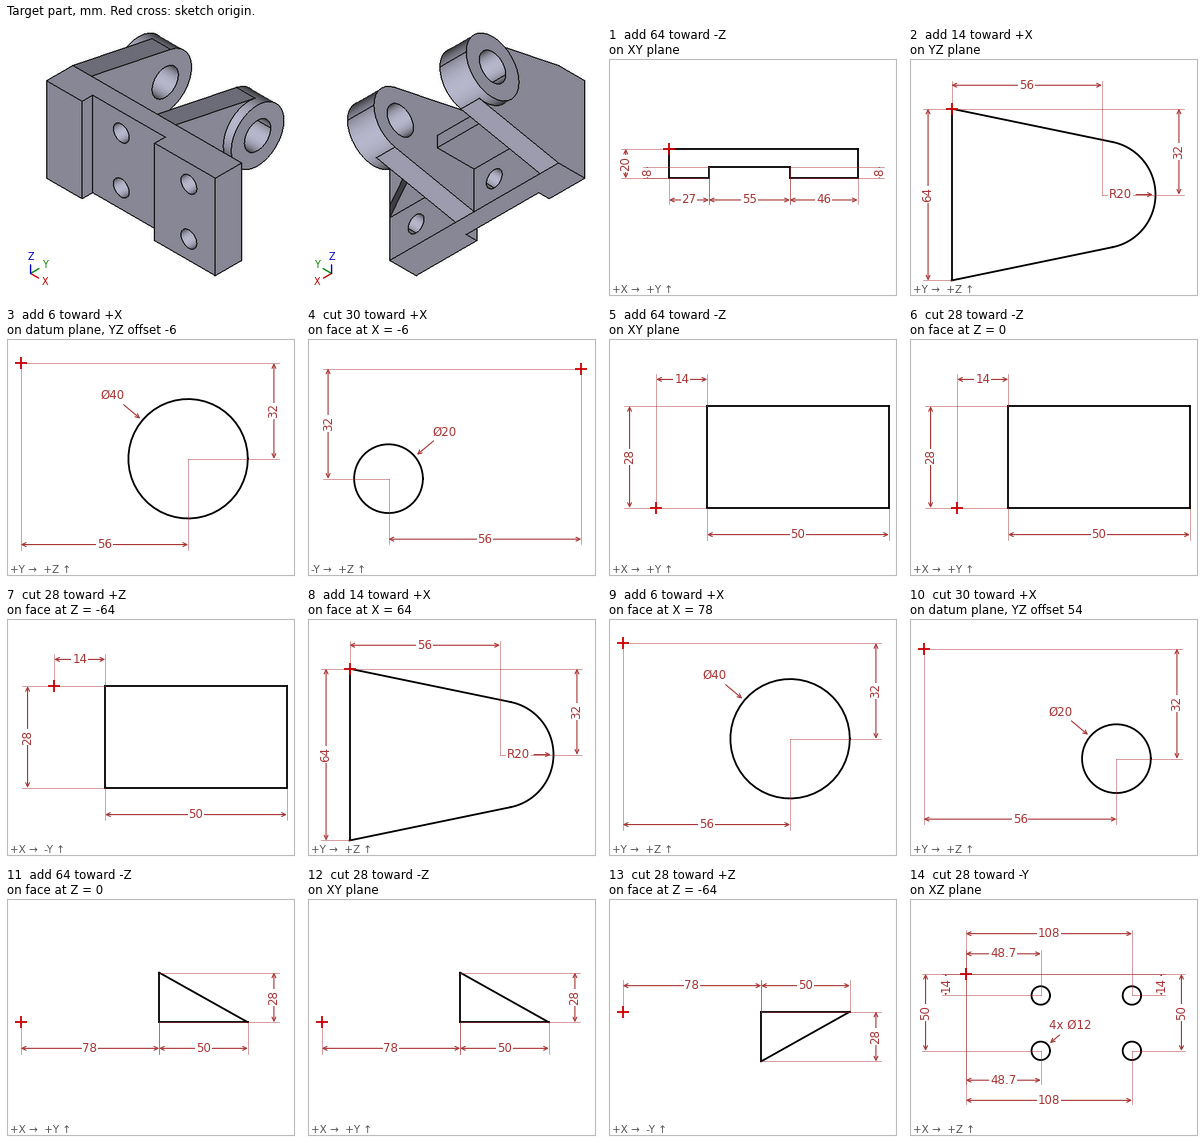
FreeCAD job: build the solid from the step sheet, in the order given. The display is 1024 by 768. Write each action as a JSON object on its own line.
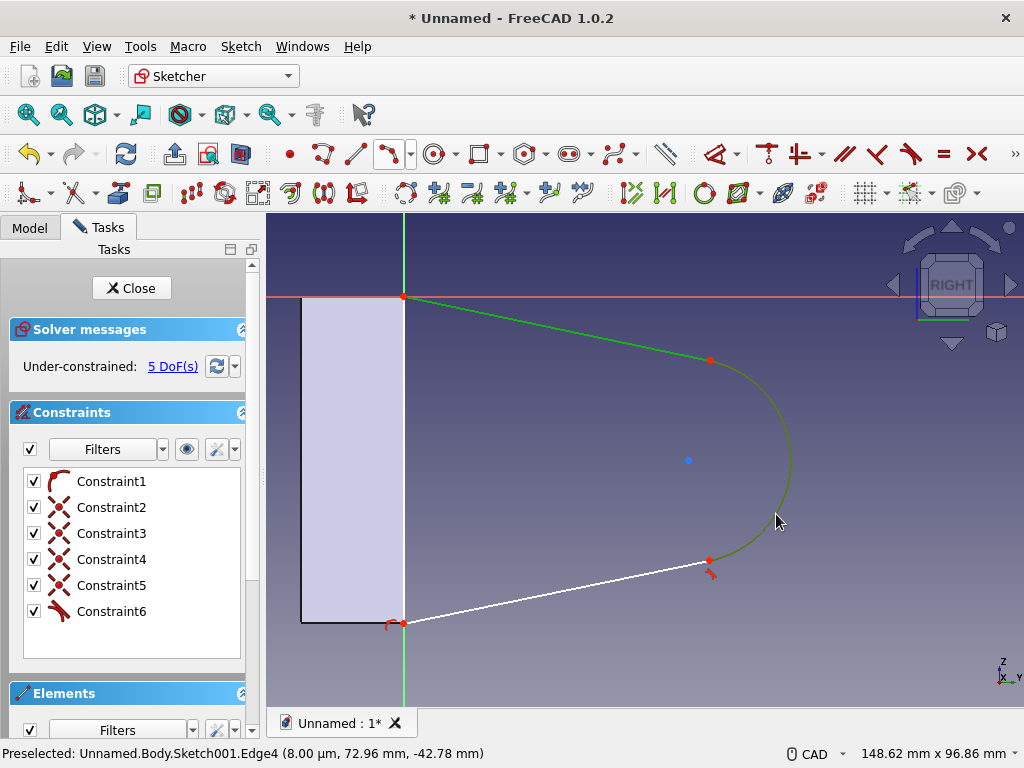
{"action": "left_click", "coordinate": [911, 154]}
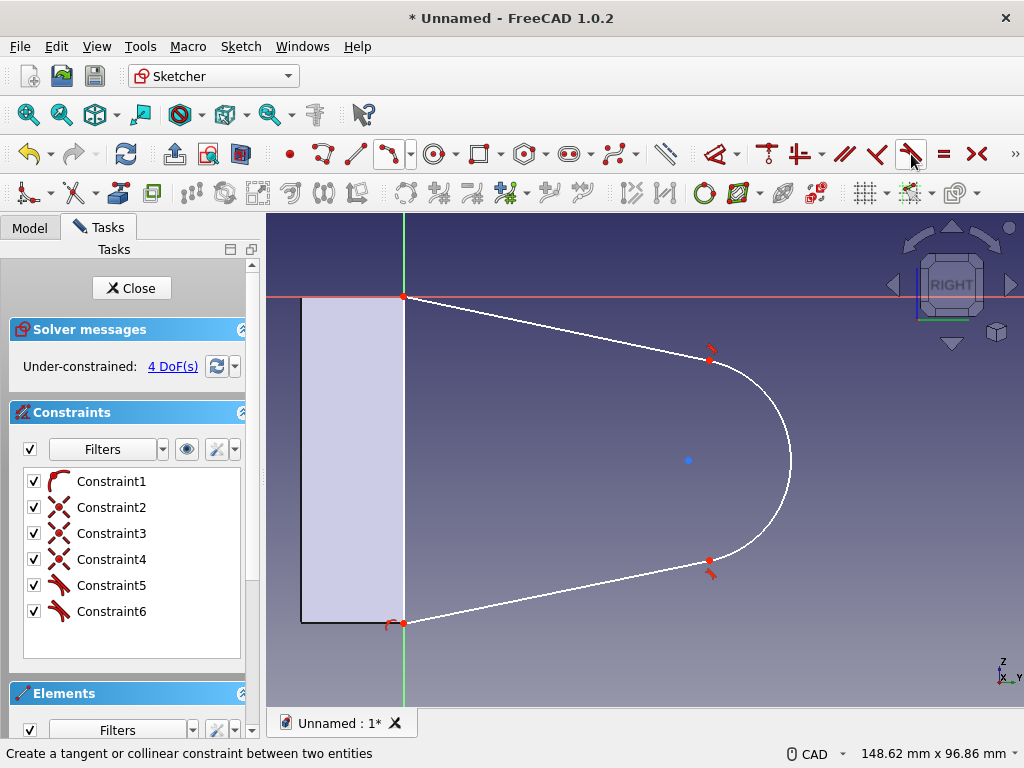
{"action": "left_click", "coordinate": [714, 154]}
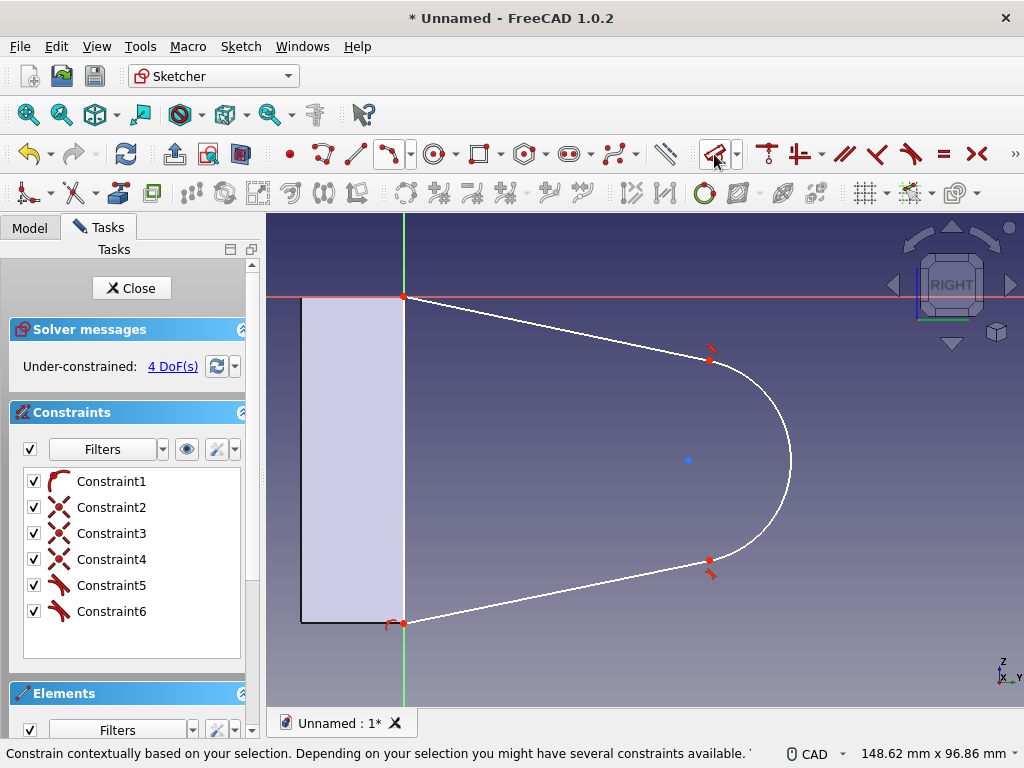
{"action": "left_click", "coordinate": [776, 514]}
{"action": "left_click", "coordinate": [803, 531]}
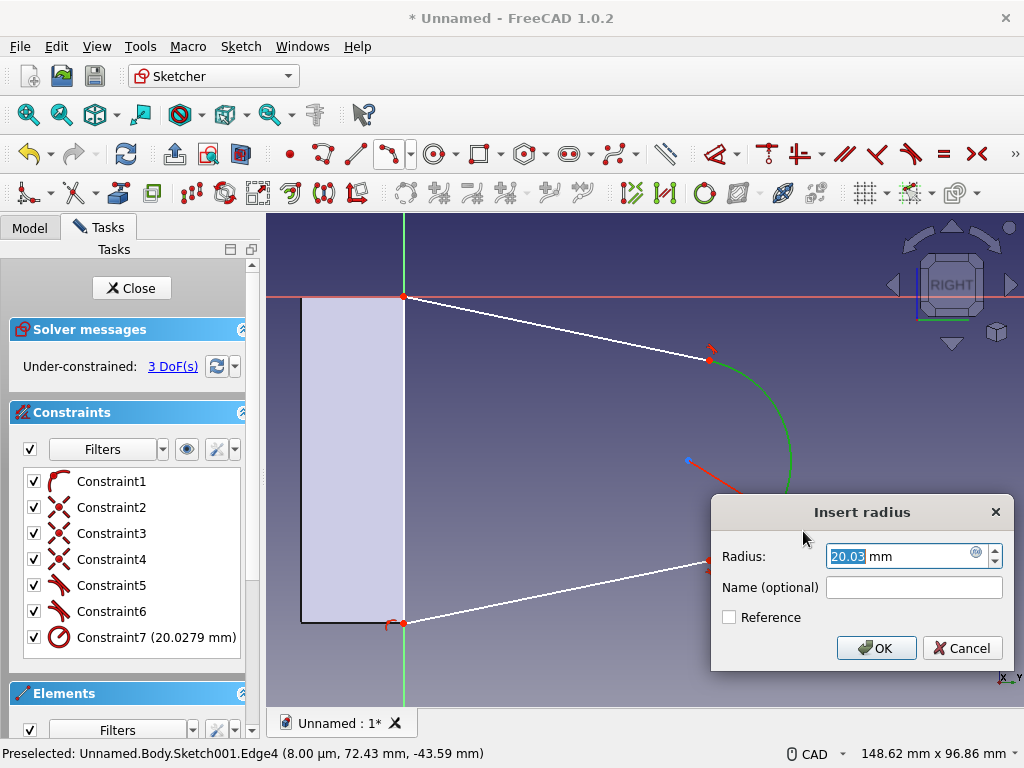
{"action": "type", "text": "20"}
{"action": "key", "text": "Return"}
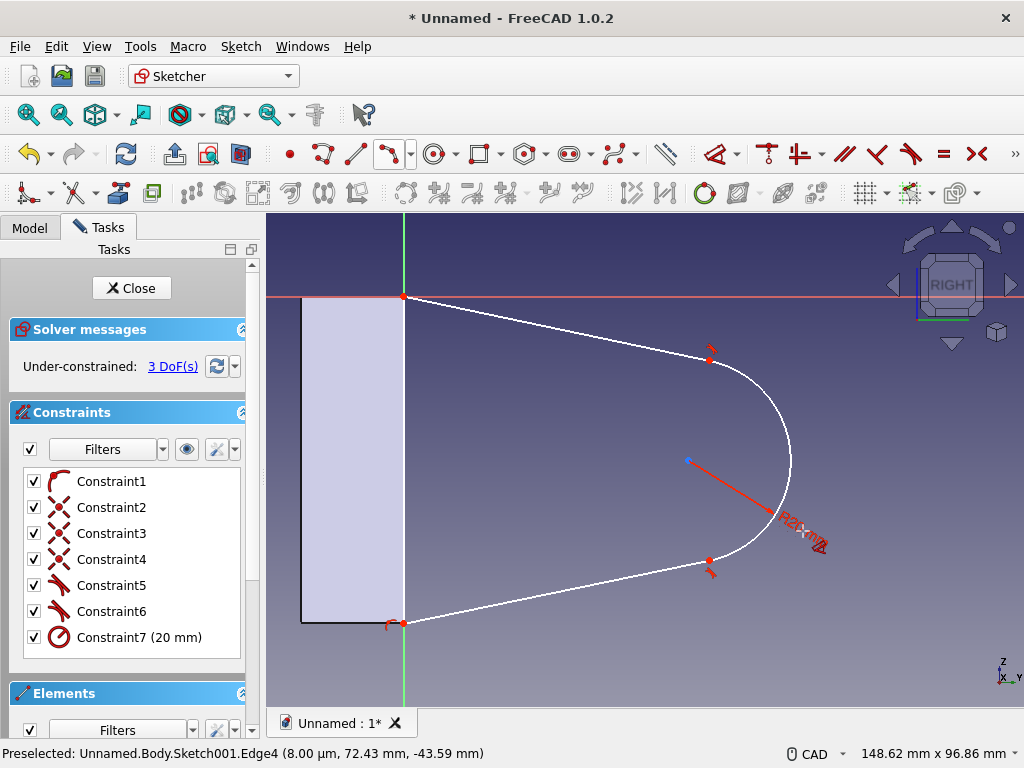
{"action": "left_click", "coordinate": [404, 526]}
{"action": "left_click", "coordinate": [370, 460]}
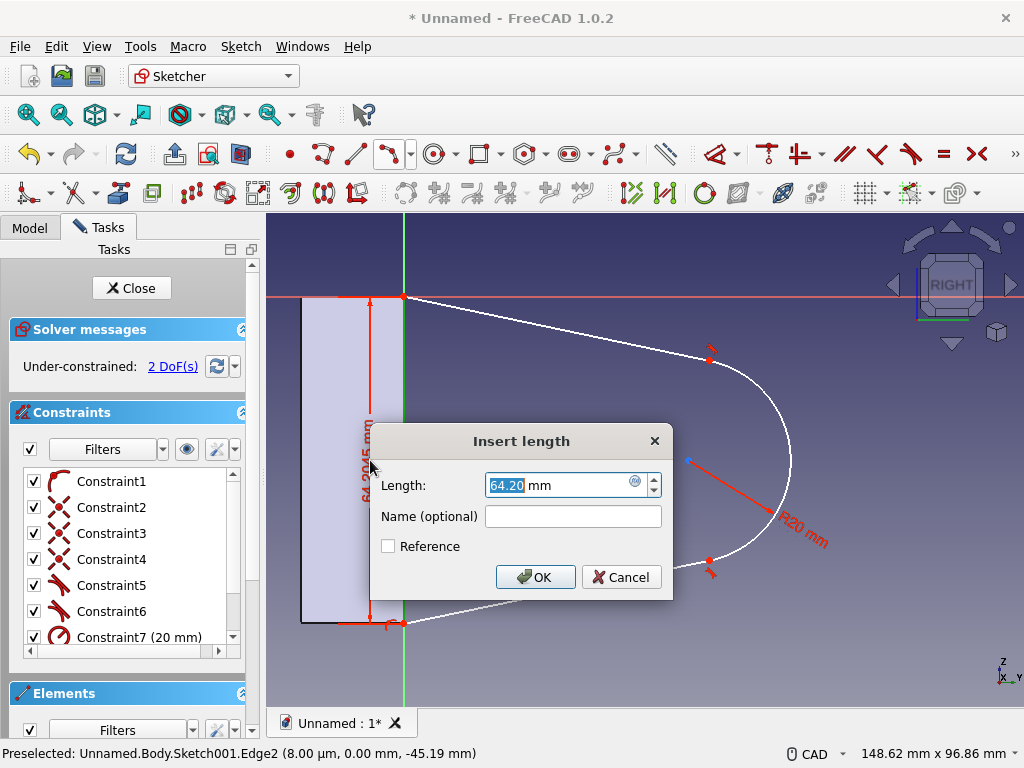
{"action": "type", "text": "64"}
{"action": "key", "text": "Return"}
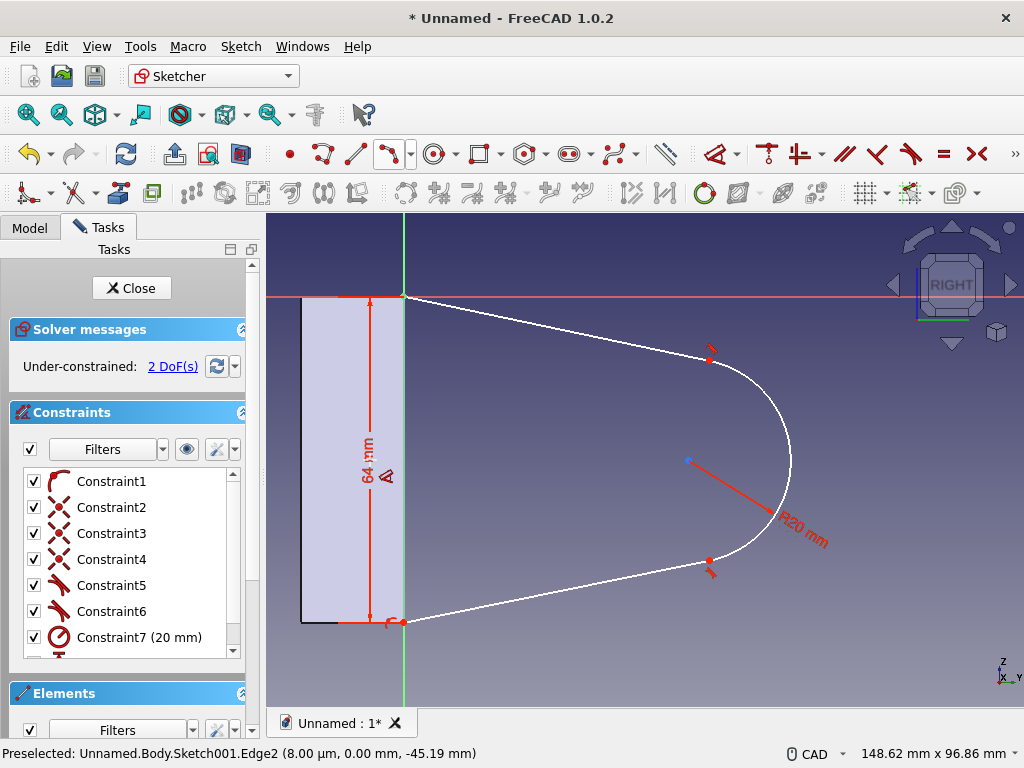
{"action": "left_click", "coordinate": [689, 461]}
{"action": "left_click", "coordinate": [546, 263]}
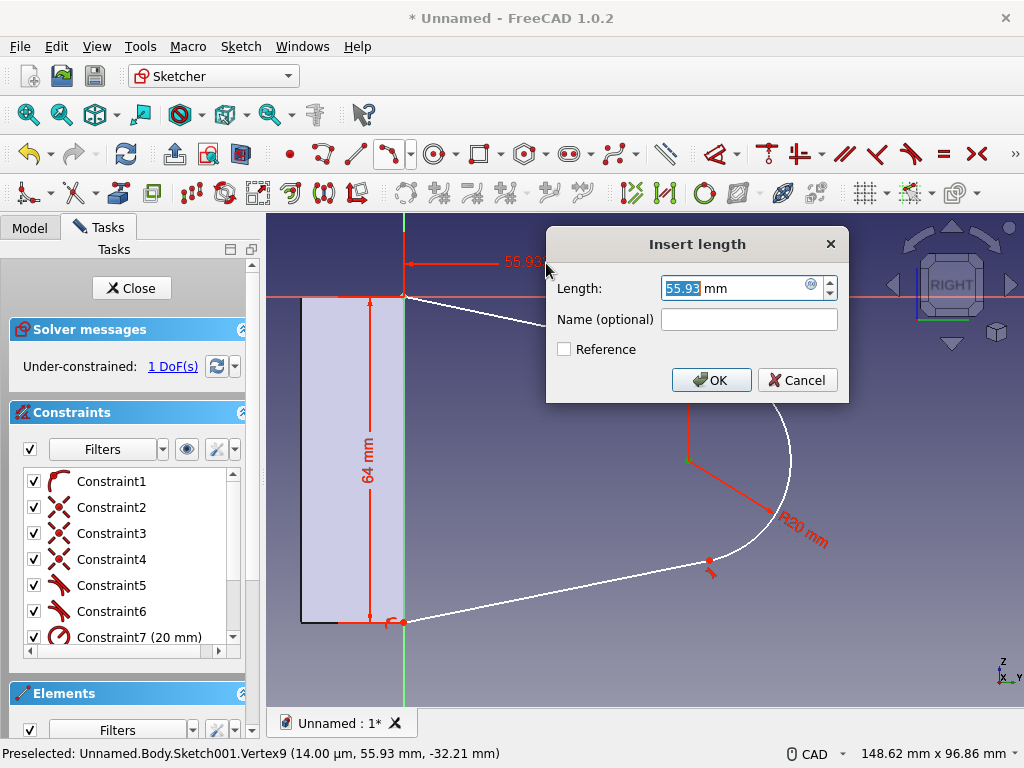
{"action": "type", "text": "56"}
{"action": "key", "text": "Return"}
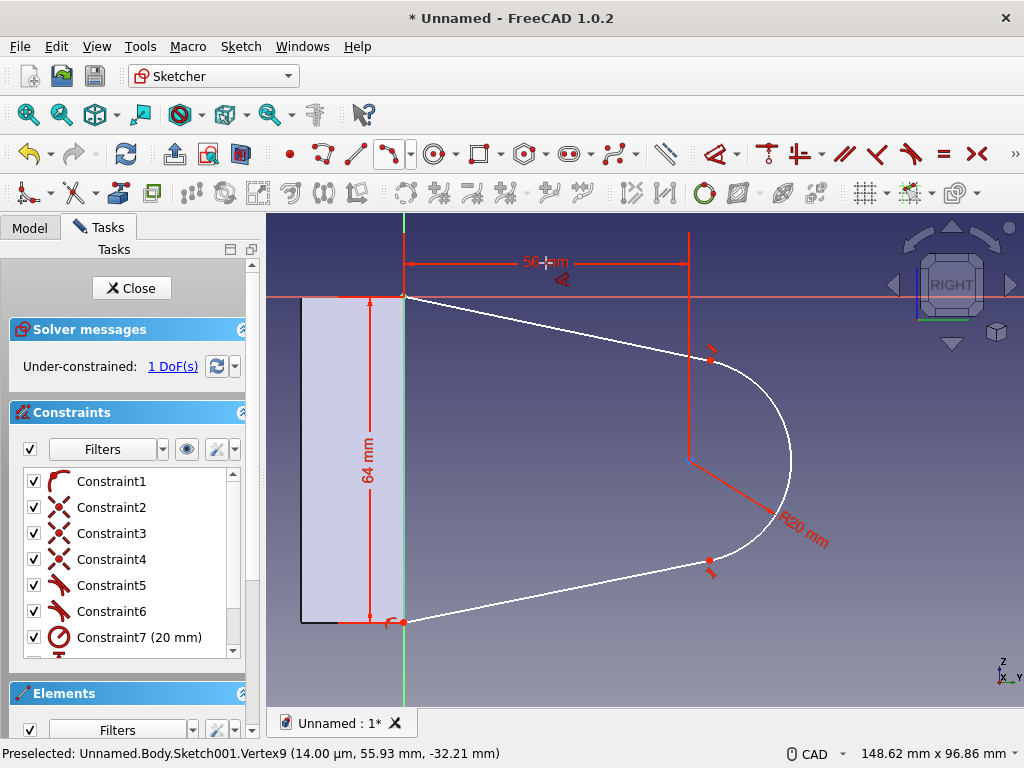
{"action": "left_click", "coordinate": [689, 461]}
{"action": "left_click", "coordinate": [370, 379]}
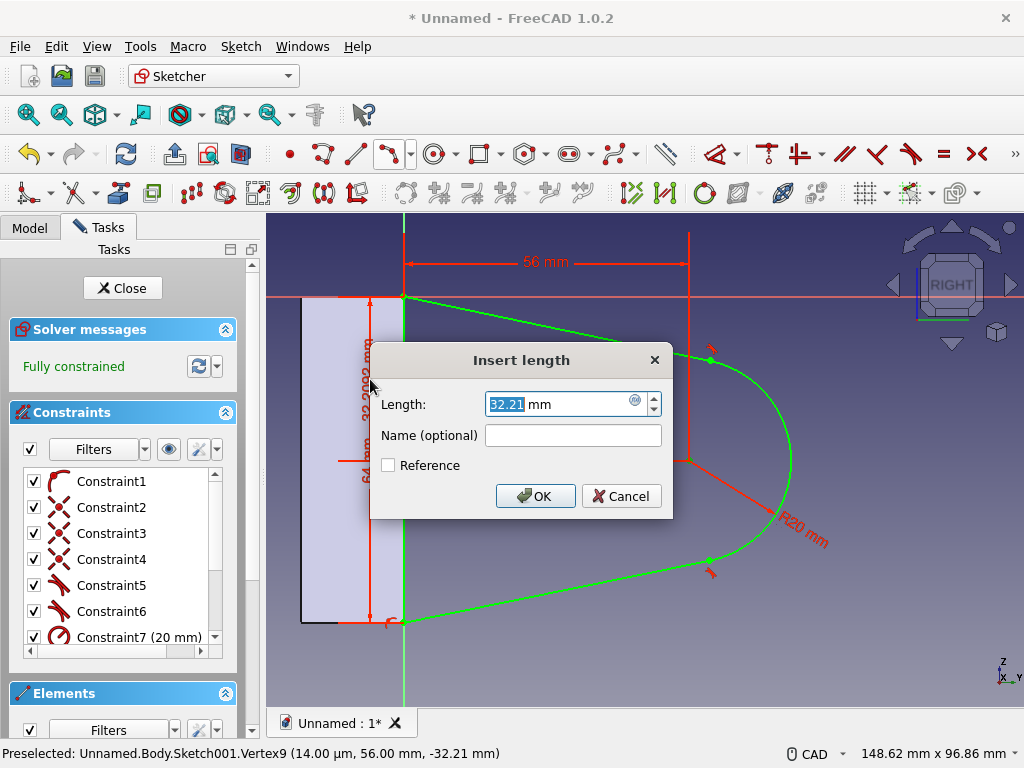
{"action": "type", "text": "32"}
{"action": "key", "text": "Return"}
{"action": "key", "text": "Escape"}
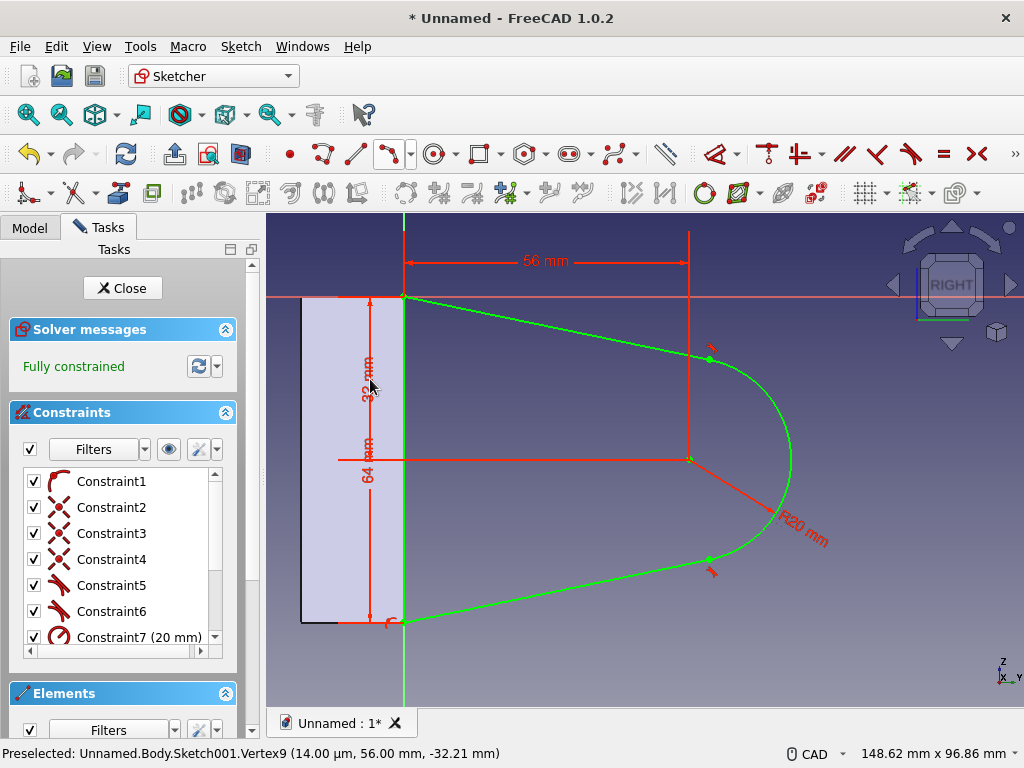
{"action": "left_click", "coordinate": [123, 288]}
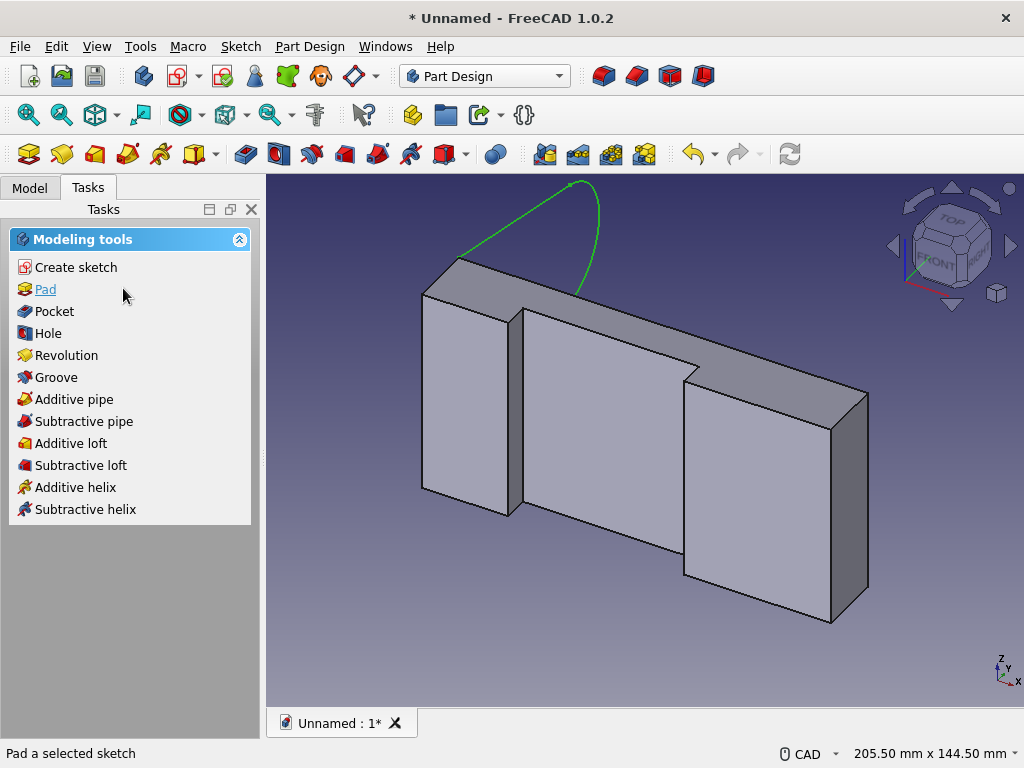
{"action": "left_click", "coordinate": [29, 154]}